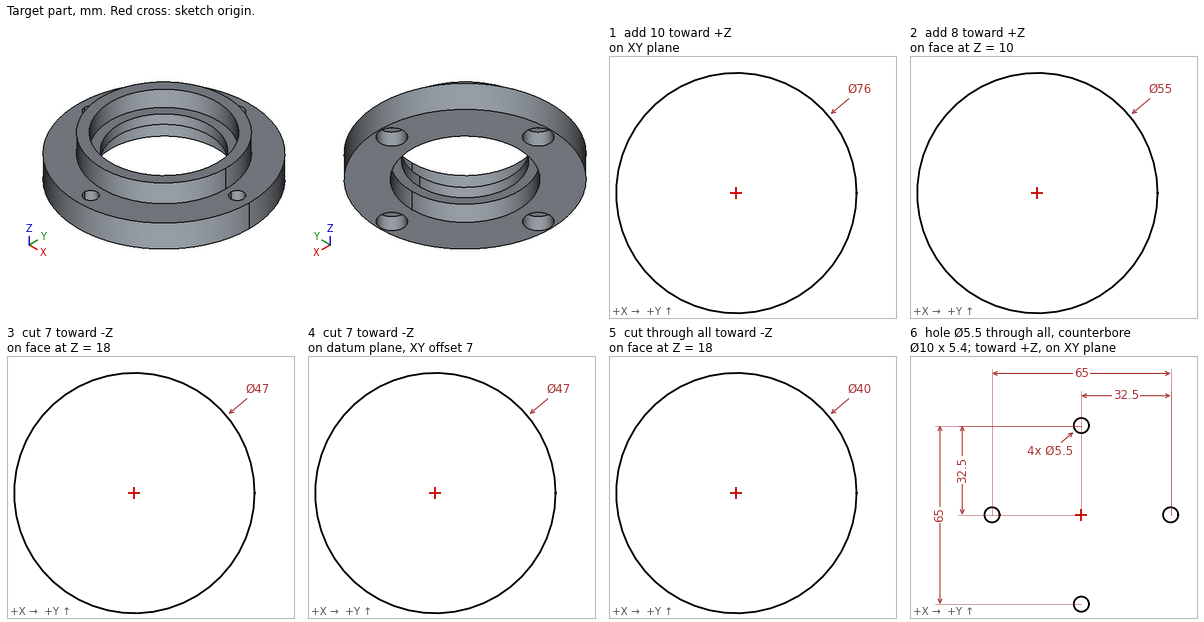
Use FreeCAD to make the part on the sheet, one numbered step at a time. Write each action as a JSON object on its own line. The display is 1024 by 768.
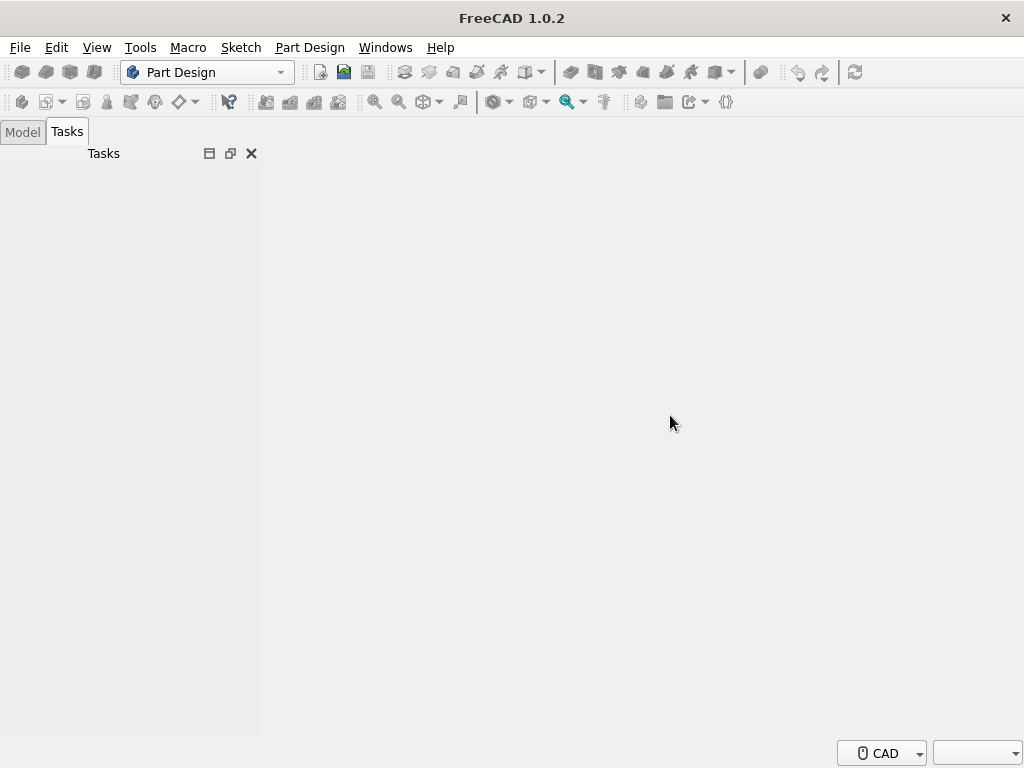
{"action": "key", "text": "ctrl+n"}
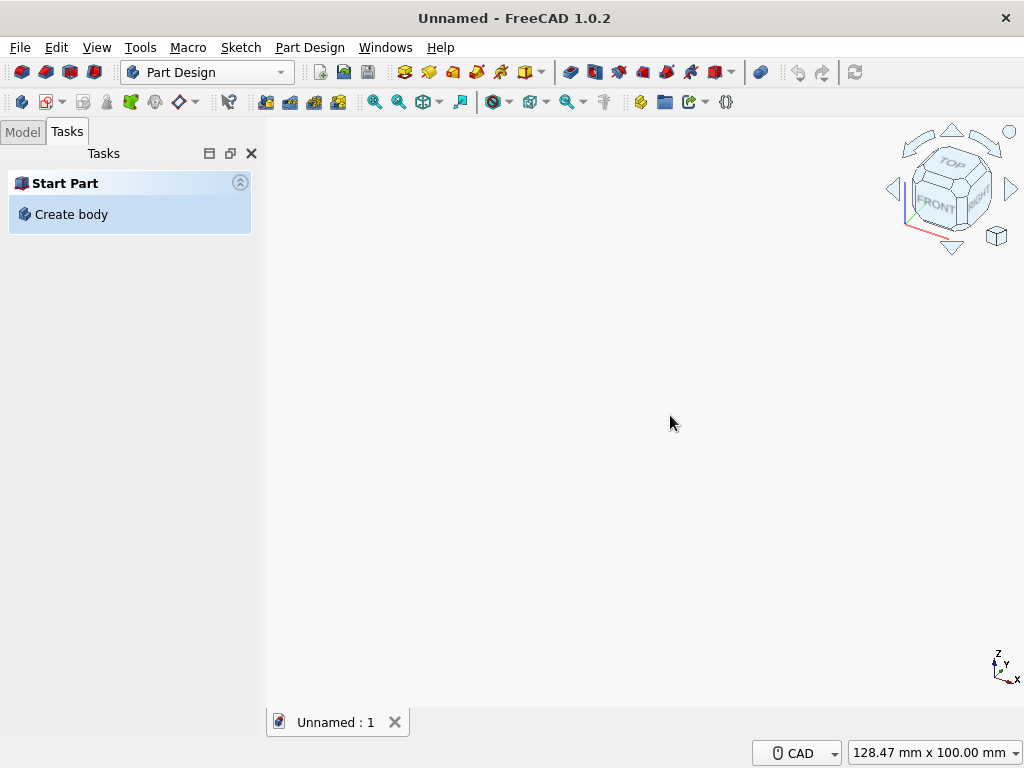
{"action": "left_click", "coordinate": [46, 102]}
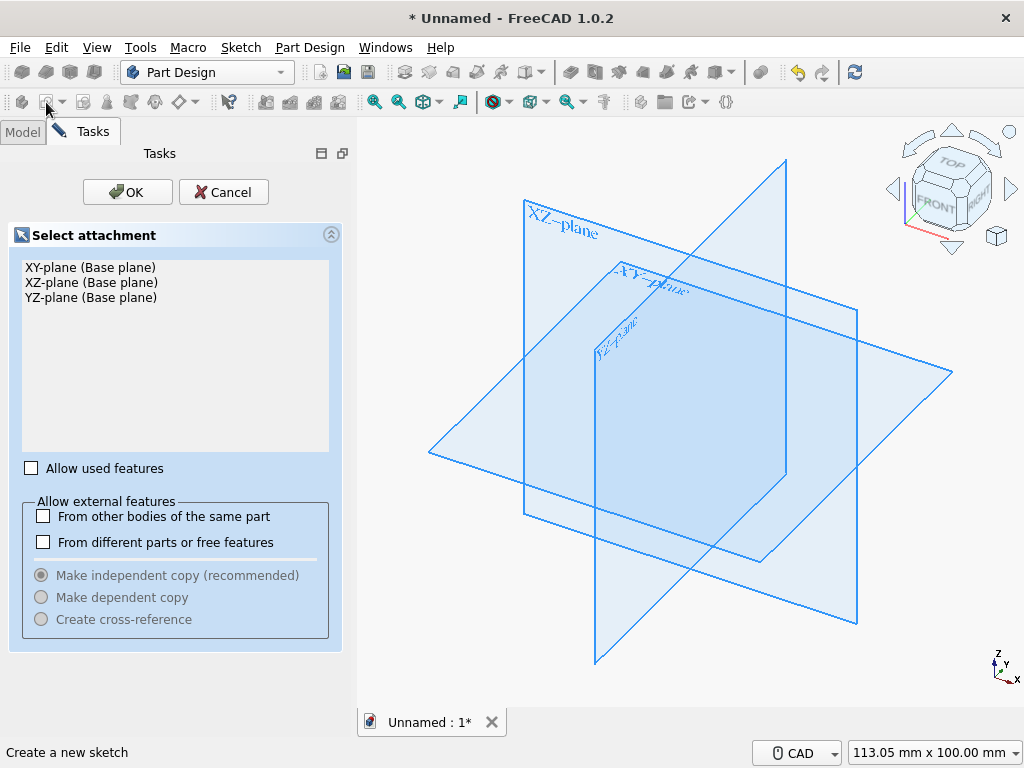
{"action": "left_click", "coordinate": [82, 268]}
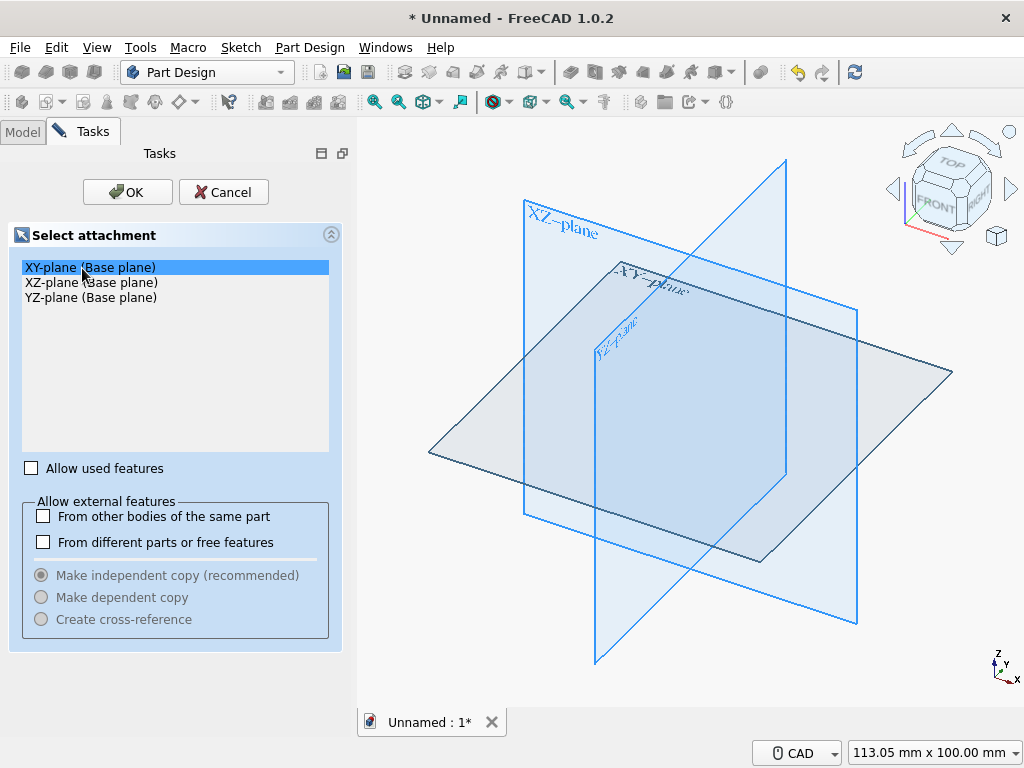
{"action": "left_click", "coordinate": [128, 192]}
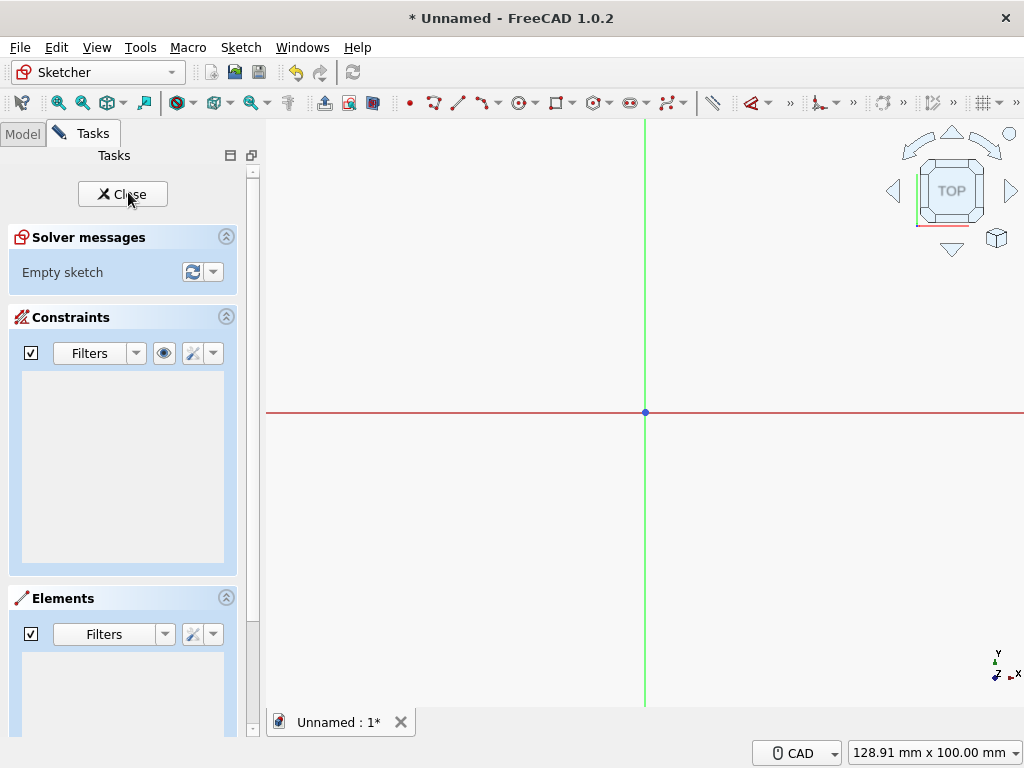
{"action": "scroll", "coordinate": [294, 413], "scroll_direction": "down", "scroll_amount": 1}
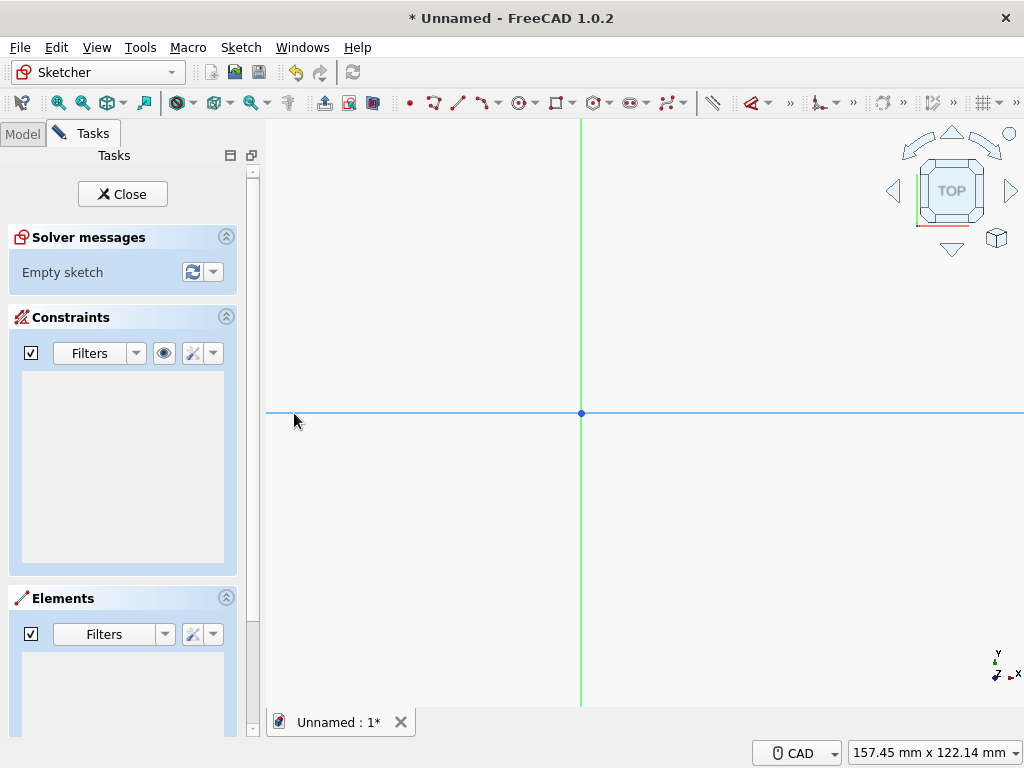
{"action": "key", "text": "g c"}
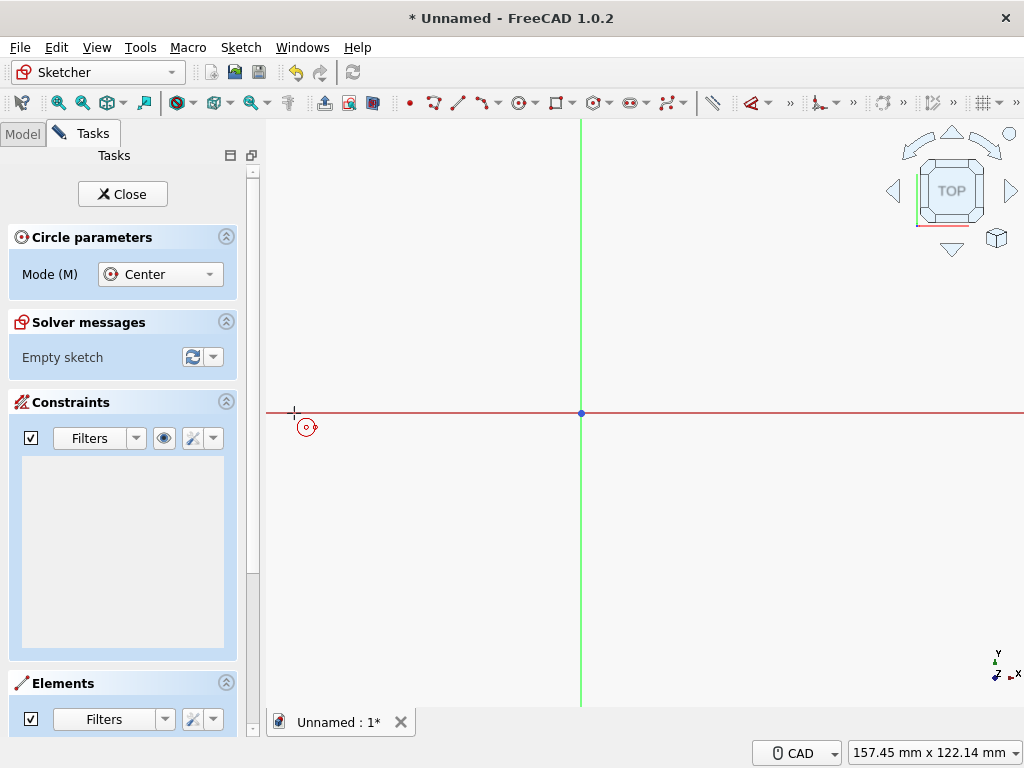
{"action": "left_click", "coordinate": [581, 413]}
{"action": "left_click", "coordinate": [711, 284]}
{"action": "key", "text": "Escape"}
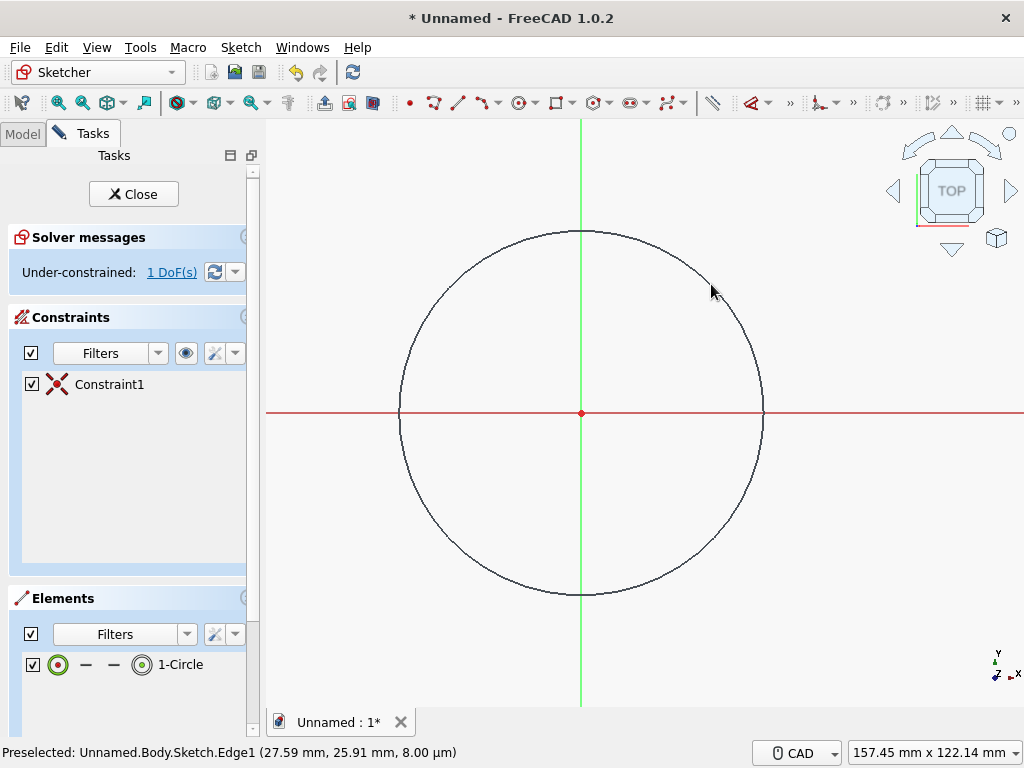
{"action": "left_click", "coordinate": [710, 284]}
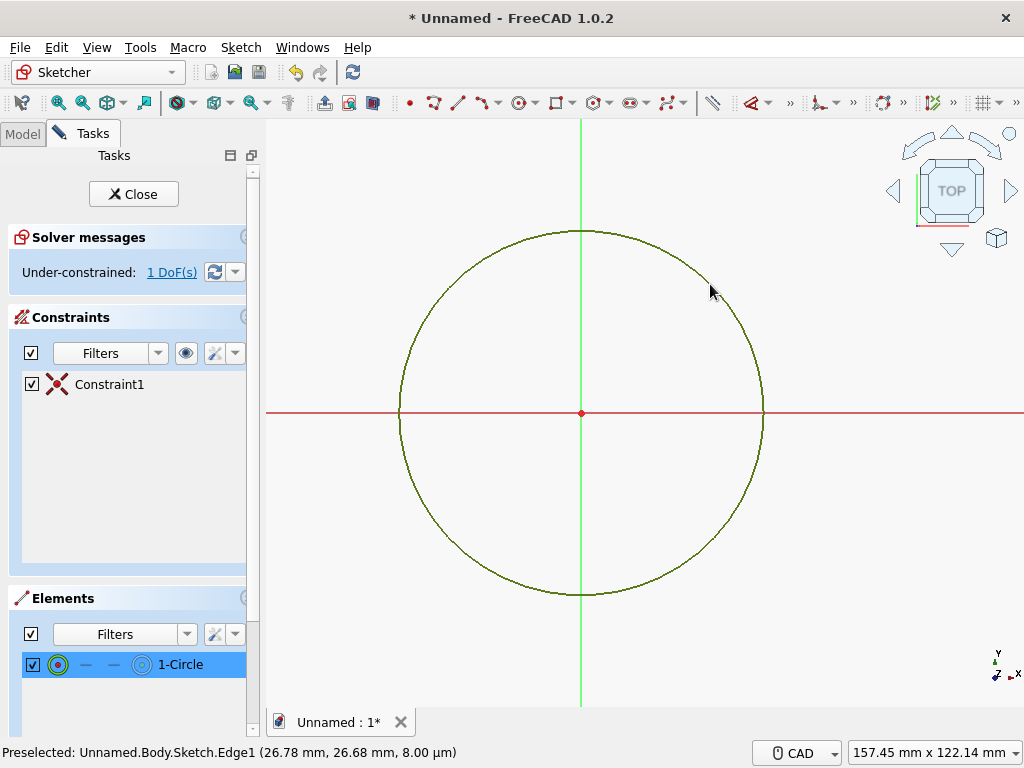
{"action": "key", "text": "k o"}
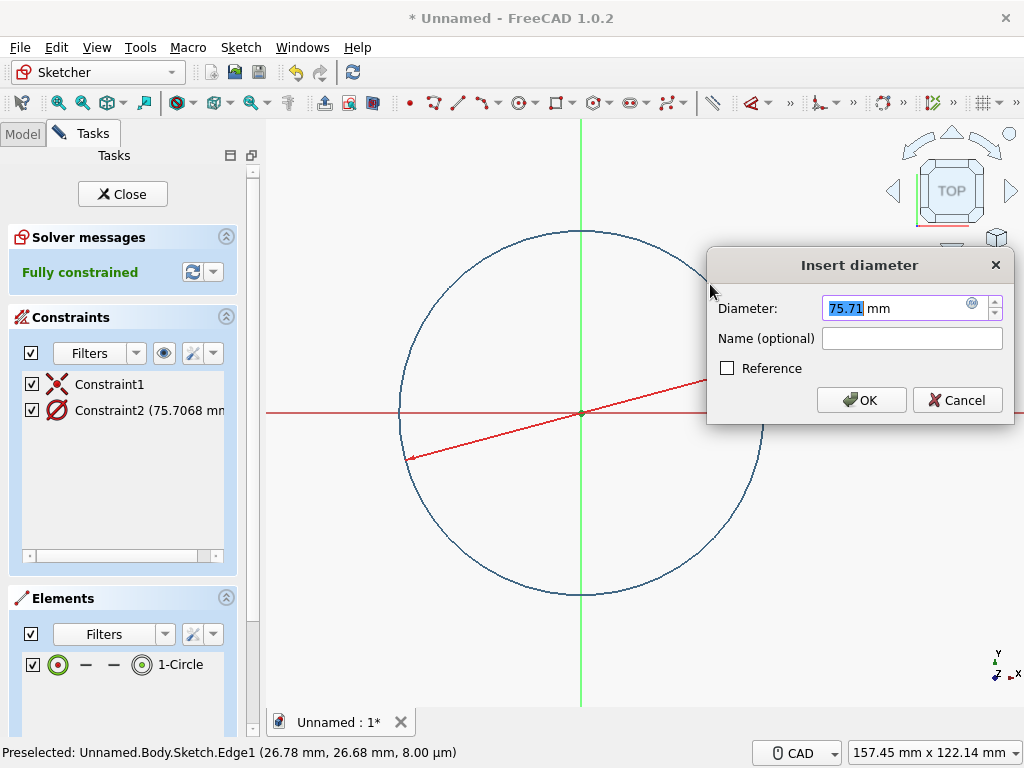
{"action": "type", "text": "76"}
{"action": "key", "text": "Return"}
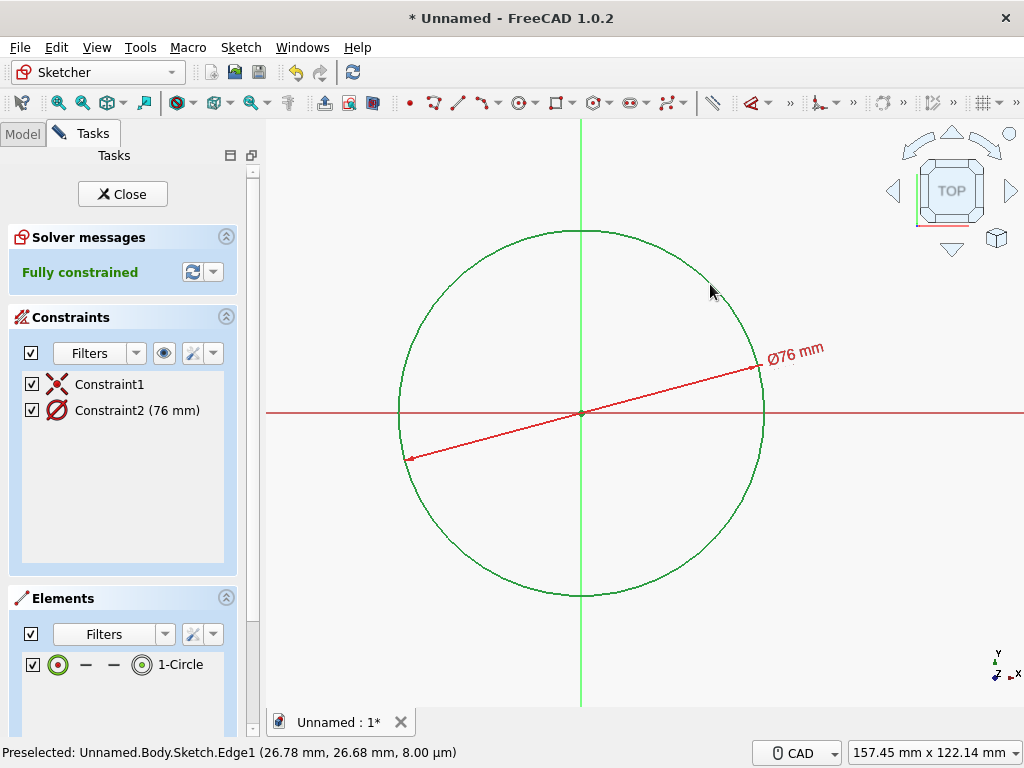
{"action": "left_click", "coordinate": [123, 194]}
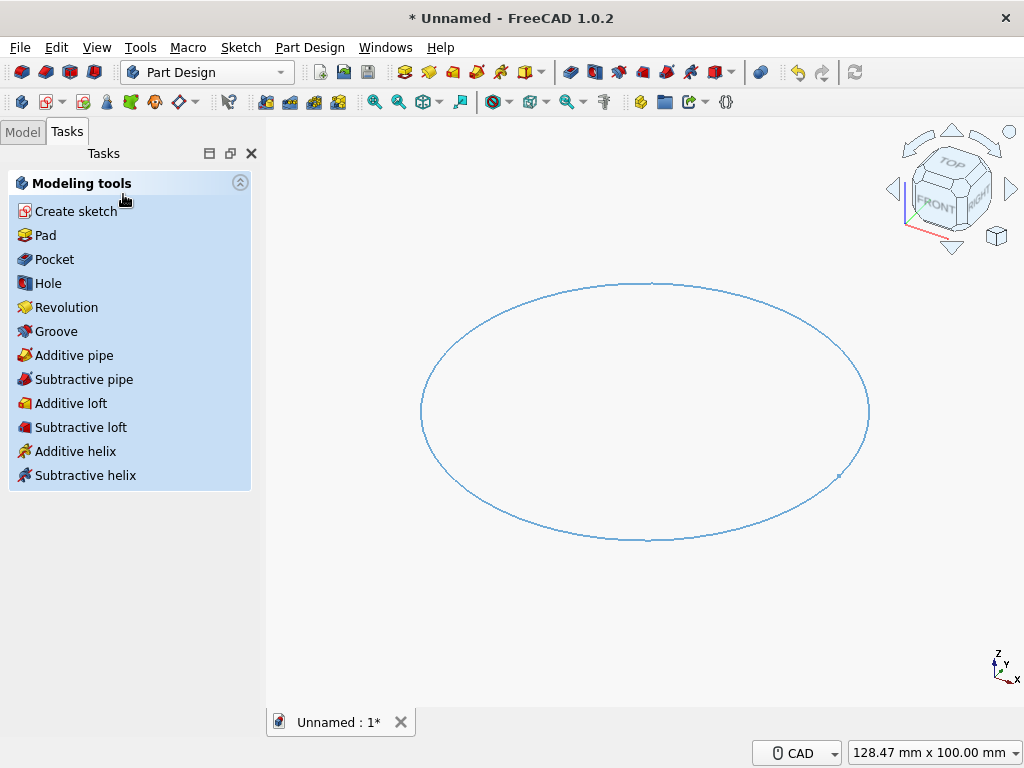
{"action": "left_click", "coordinate": [406, 72]}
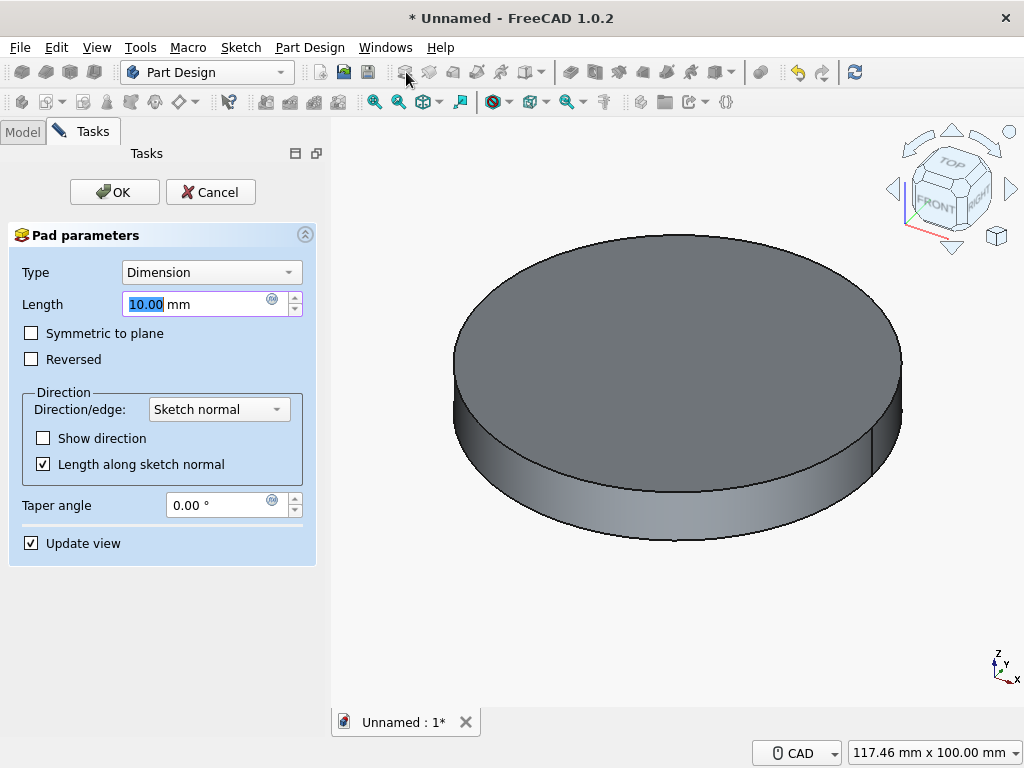
{"action": "type", "text": "10"}
{"action": "key", "text": "Tab"}